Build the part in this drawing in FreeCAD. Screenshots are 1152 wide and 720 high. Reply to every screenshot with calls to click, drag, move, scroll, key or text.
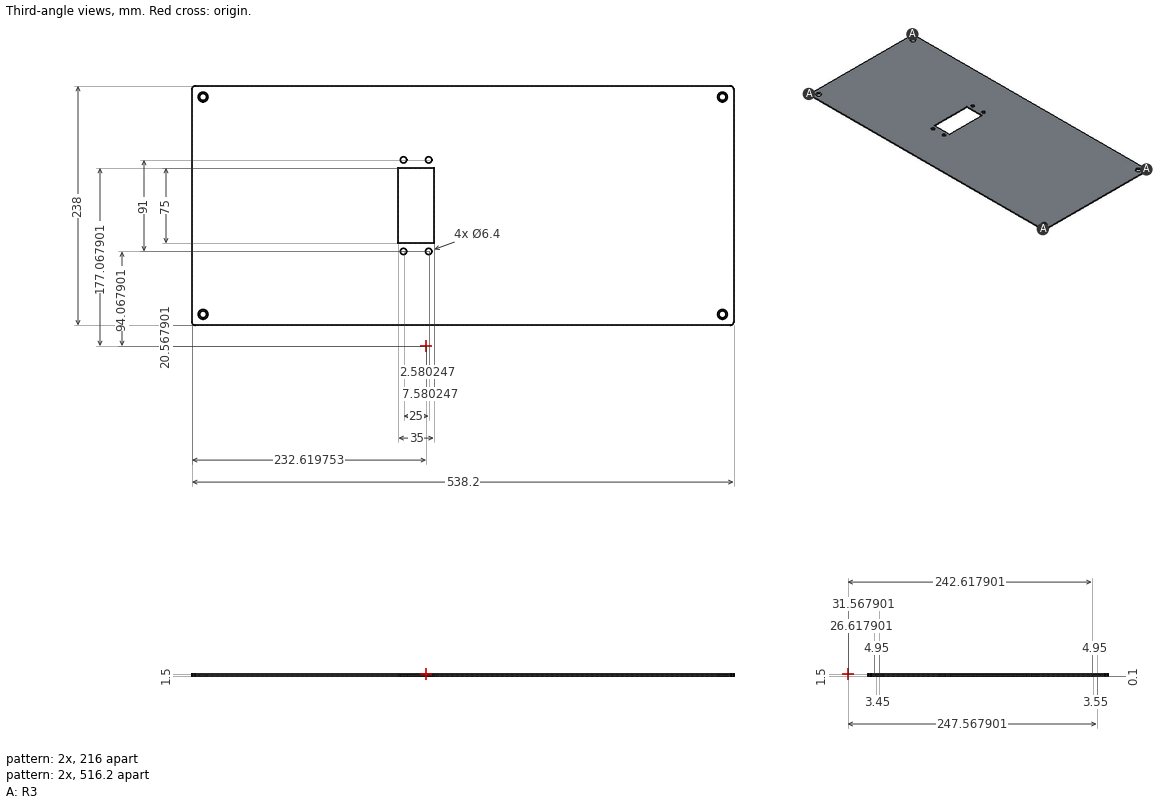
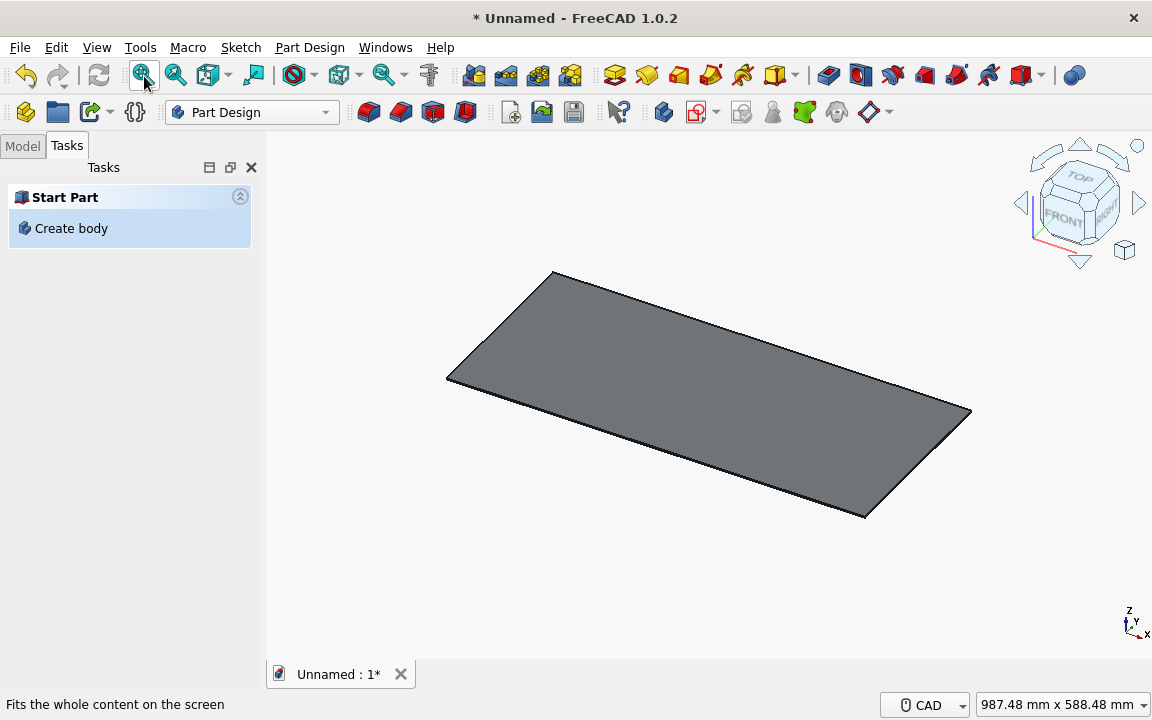
click(23, 145)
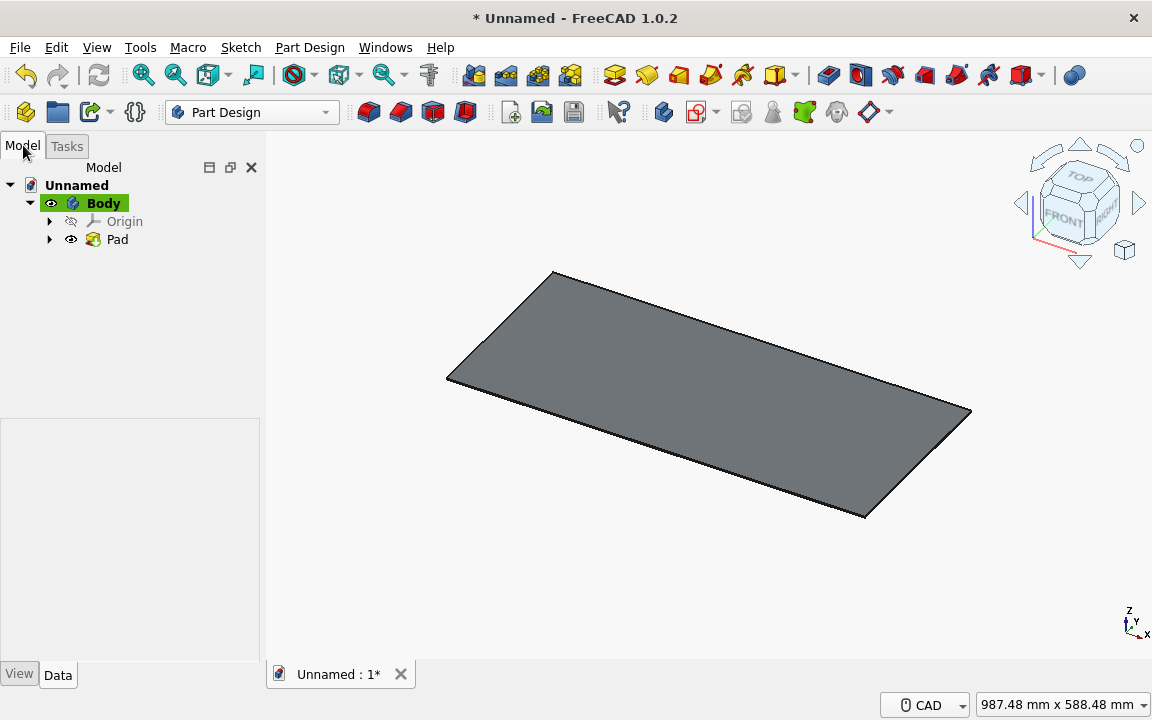
click(50, 221)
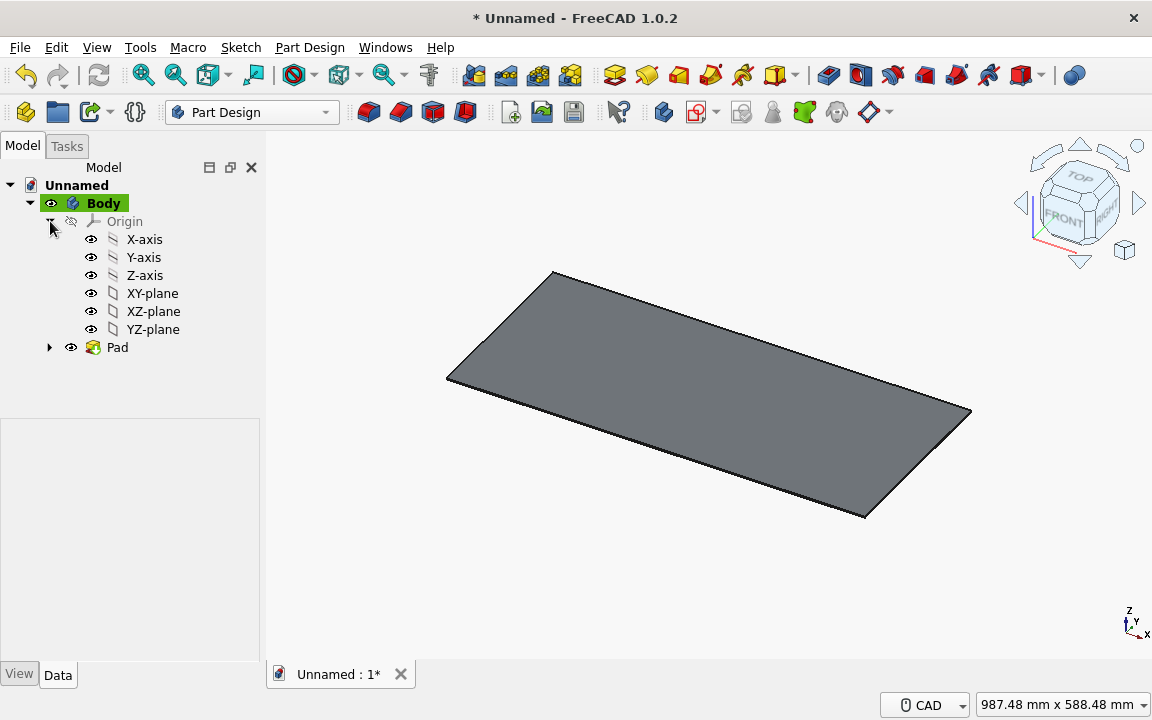
click(136, 329)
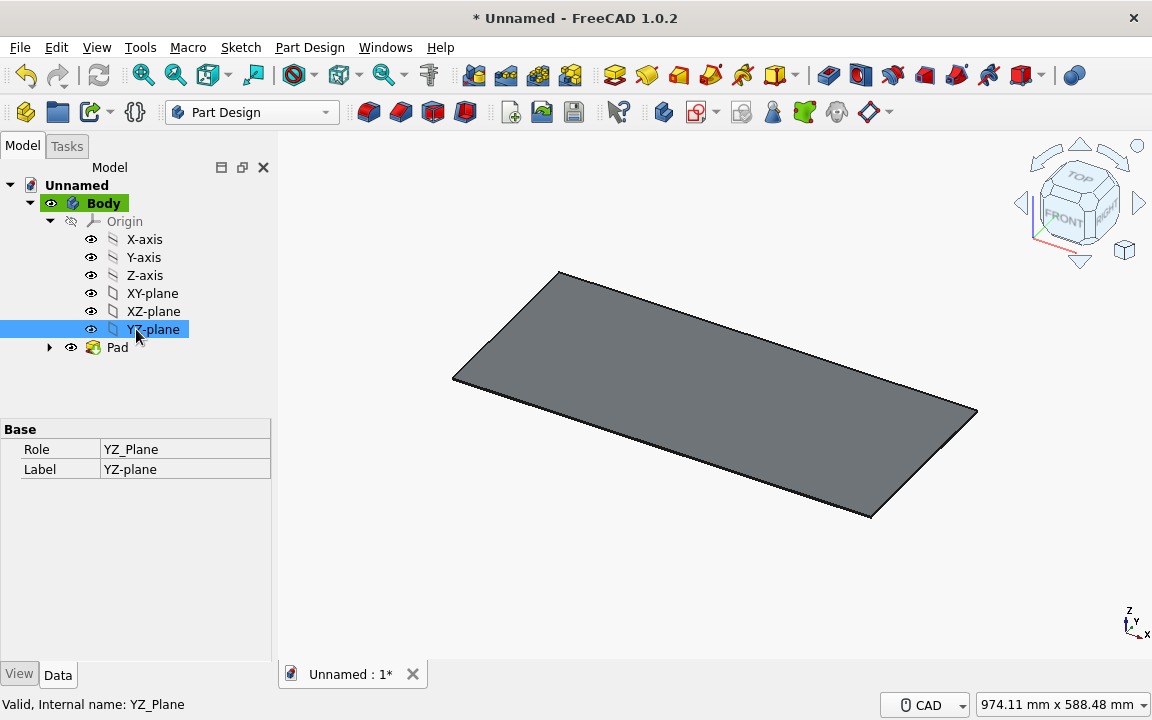
click(870, 112)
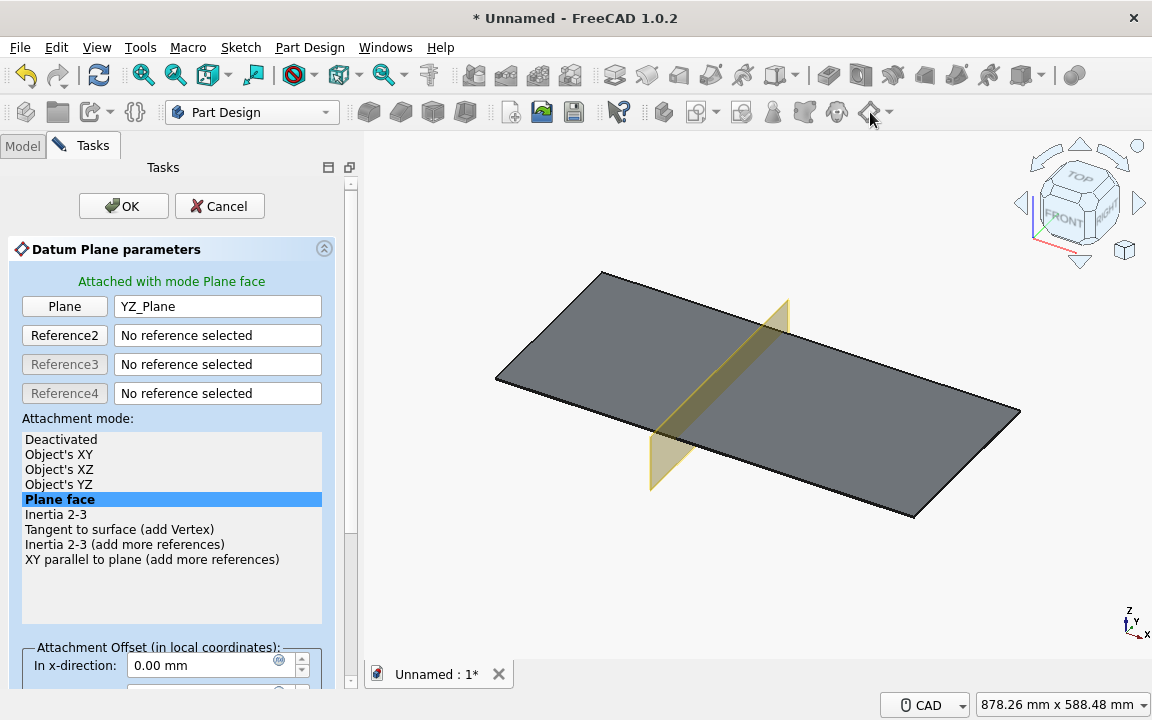
scroll(351, 432, down, 2)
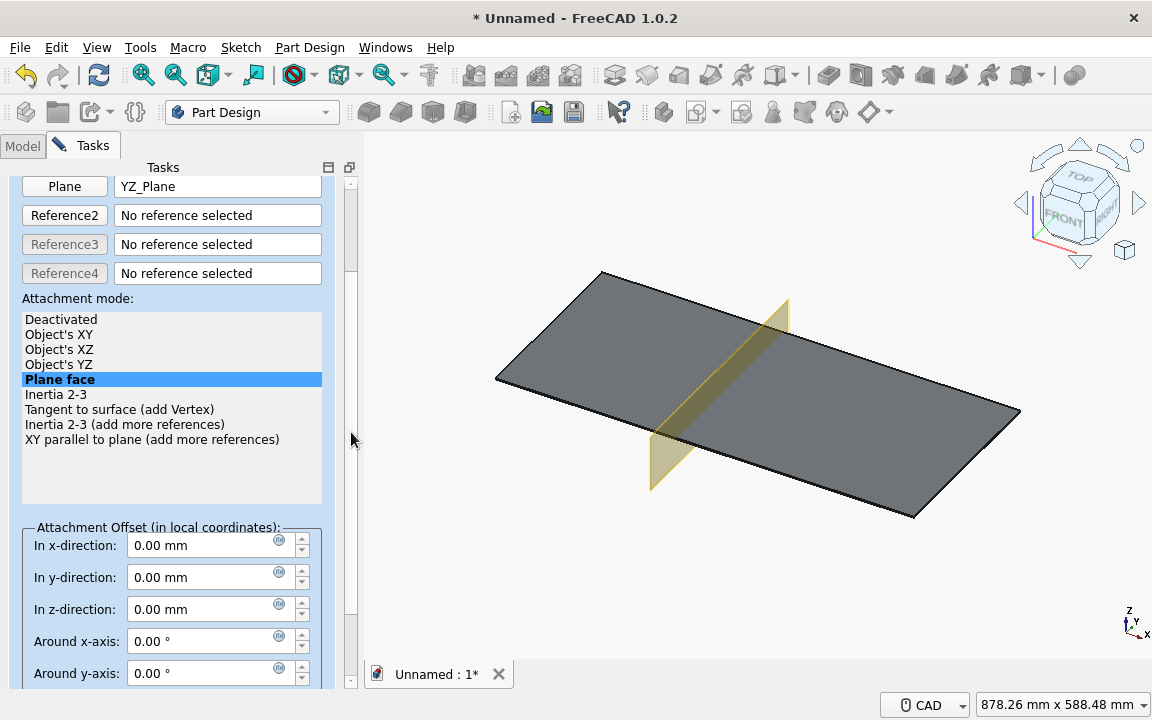
triple_click(210, 609)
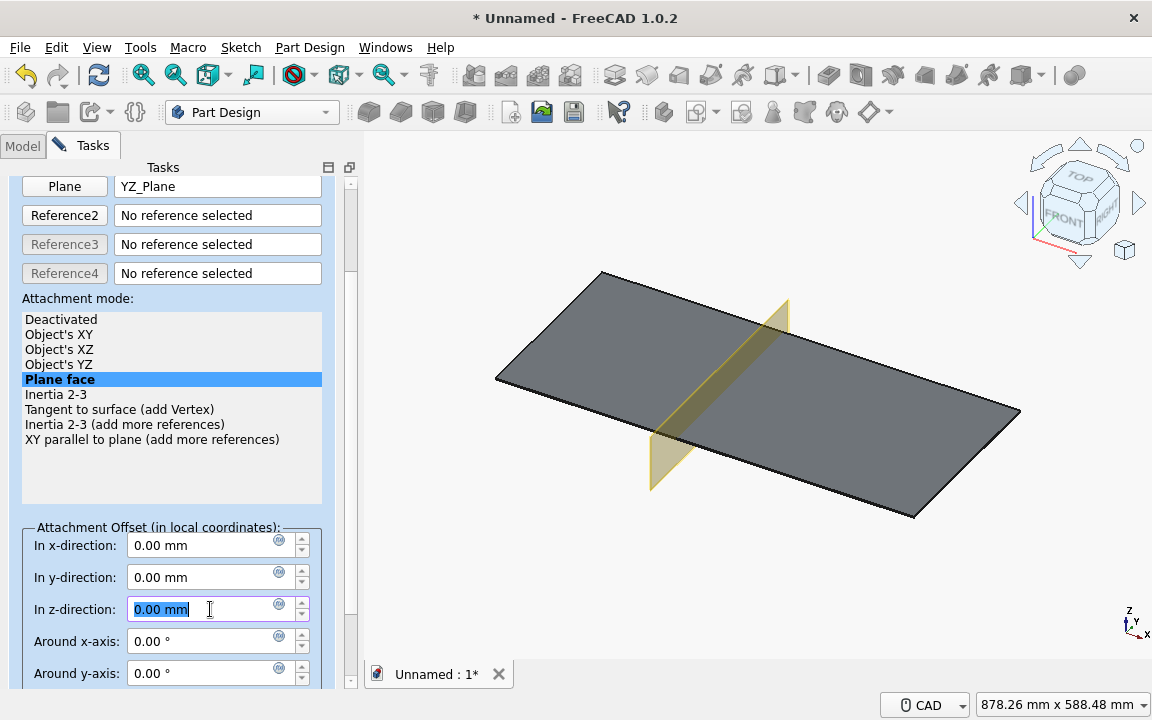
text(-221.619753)
key(Tab)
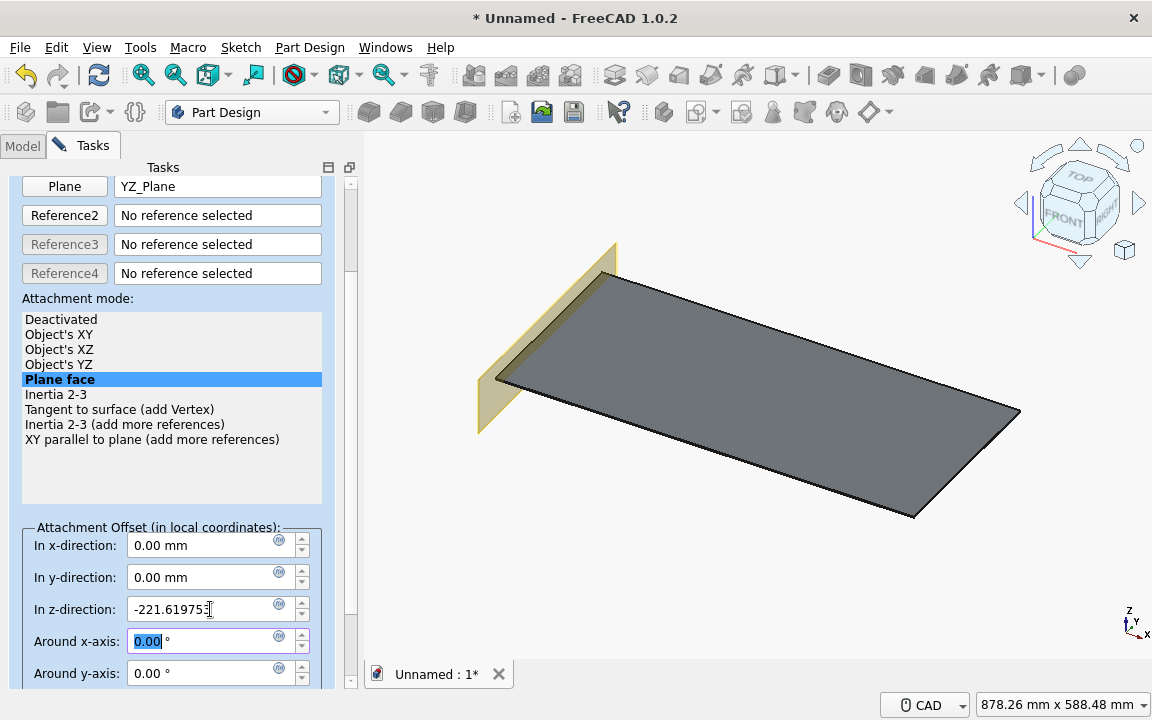
scroll(351, 432, up, 3)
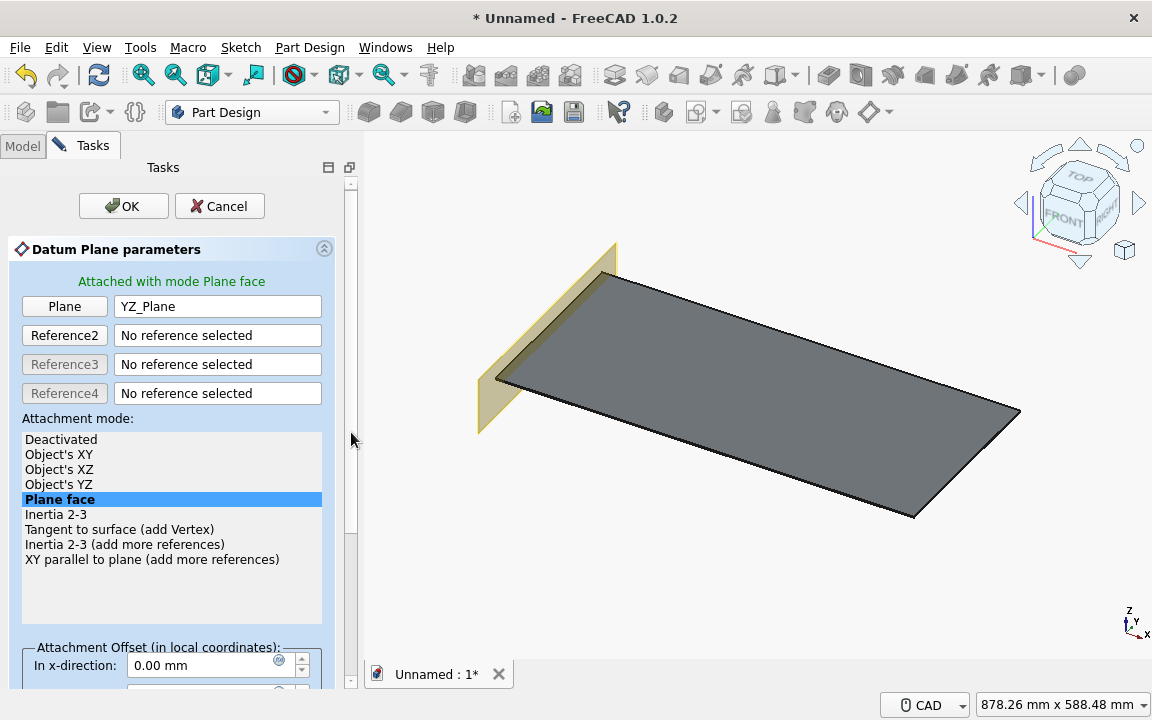
click(124, 206)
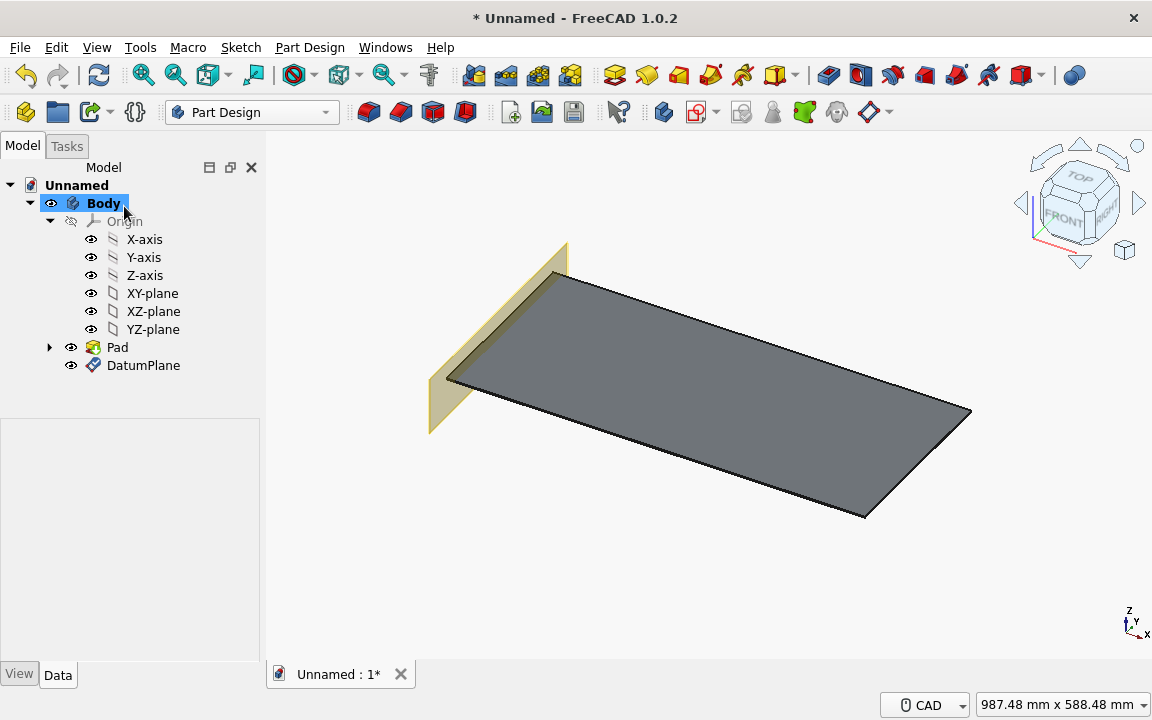
click(116, 365)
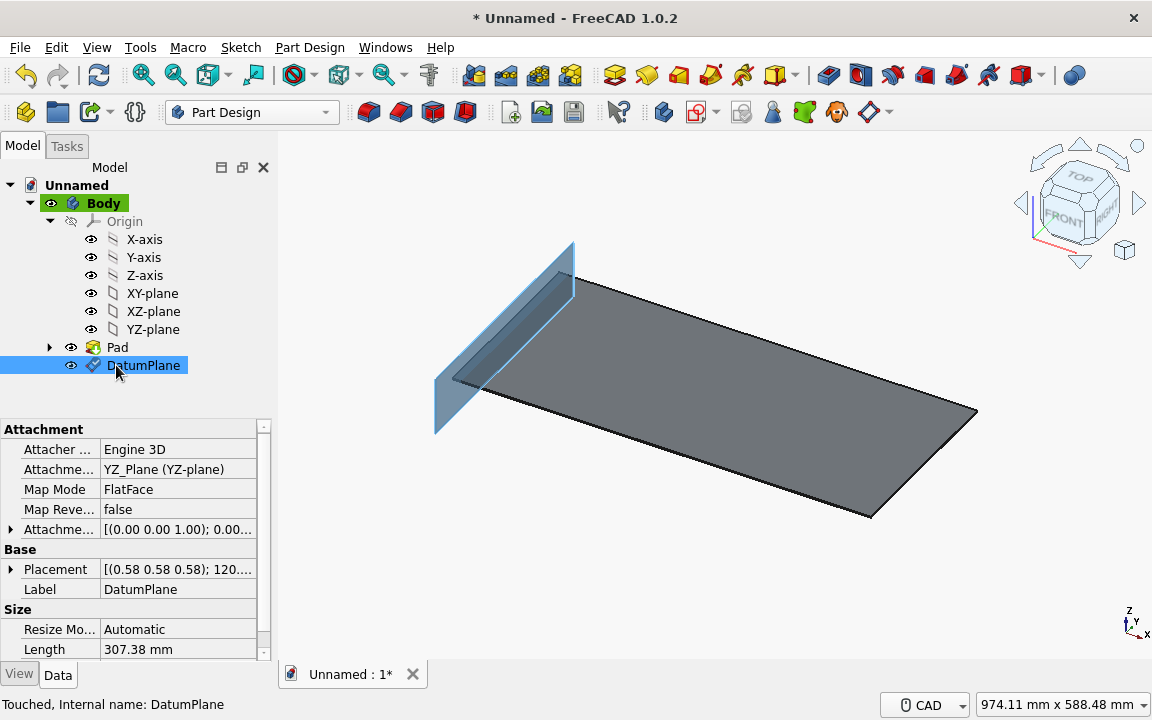
click(696, 112)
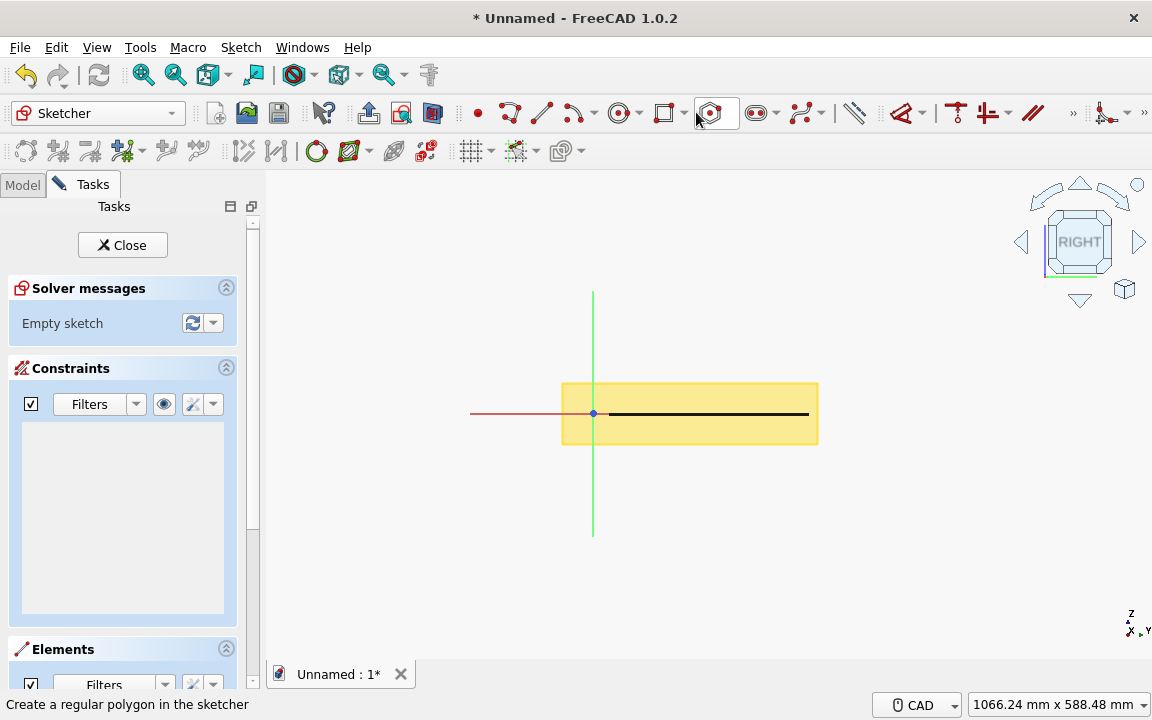
key(q)
key(s)